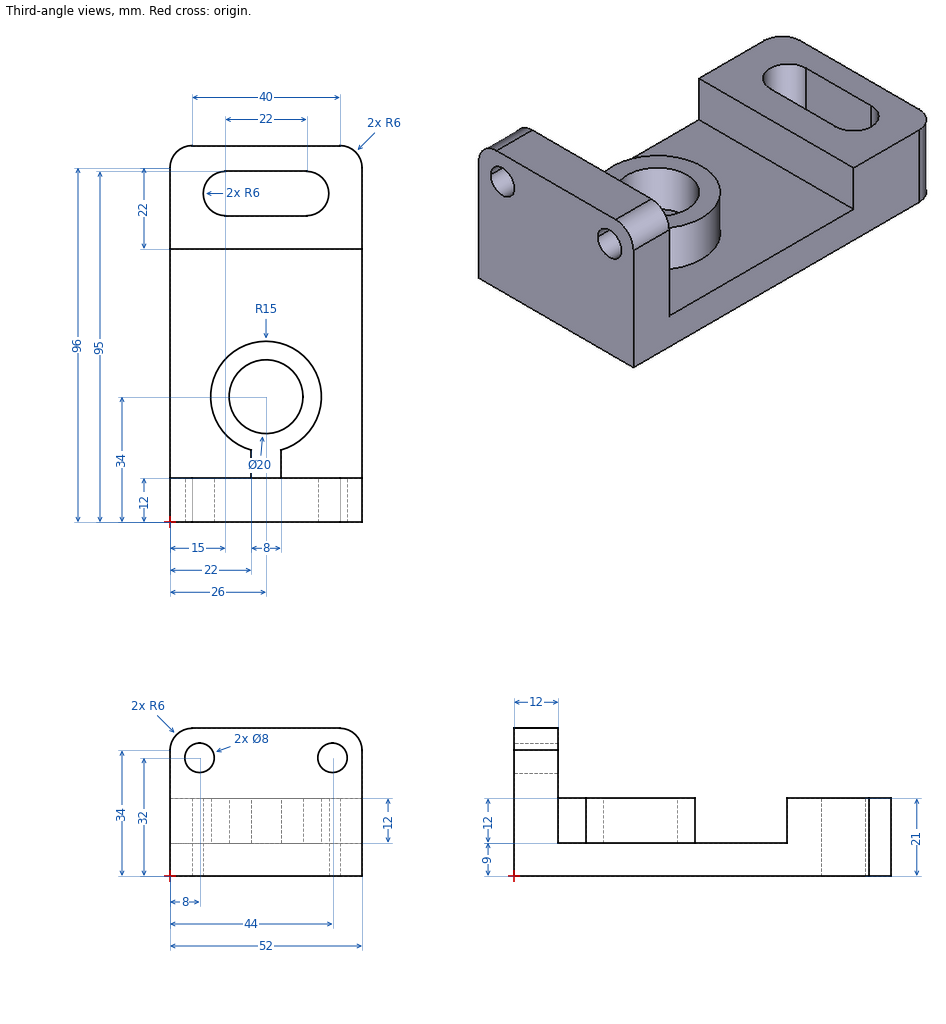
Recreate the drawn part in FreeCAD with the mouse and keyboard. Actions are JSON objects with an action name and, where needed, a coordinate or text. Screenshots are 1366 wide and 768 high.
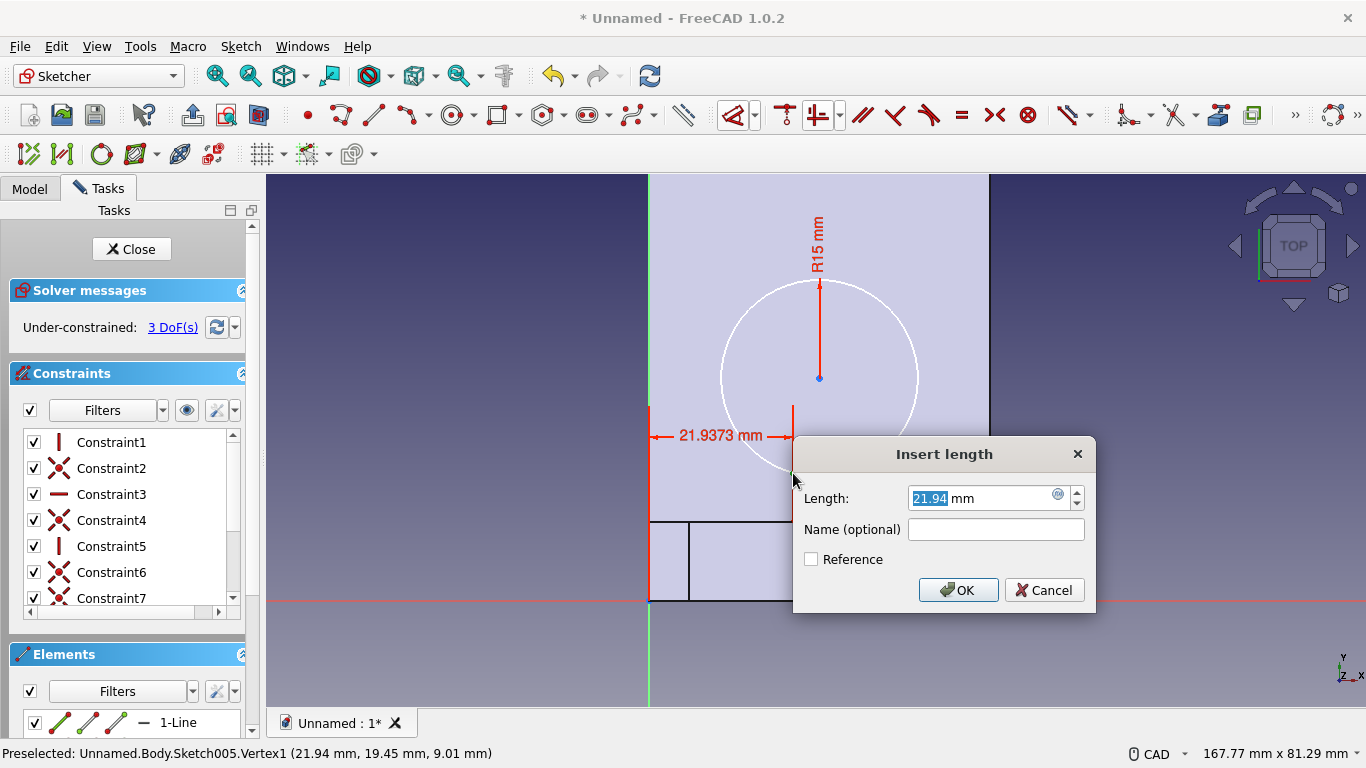
{"action": "type", "text": "22"}
{"action": "key", "text": "Return"}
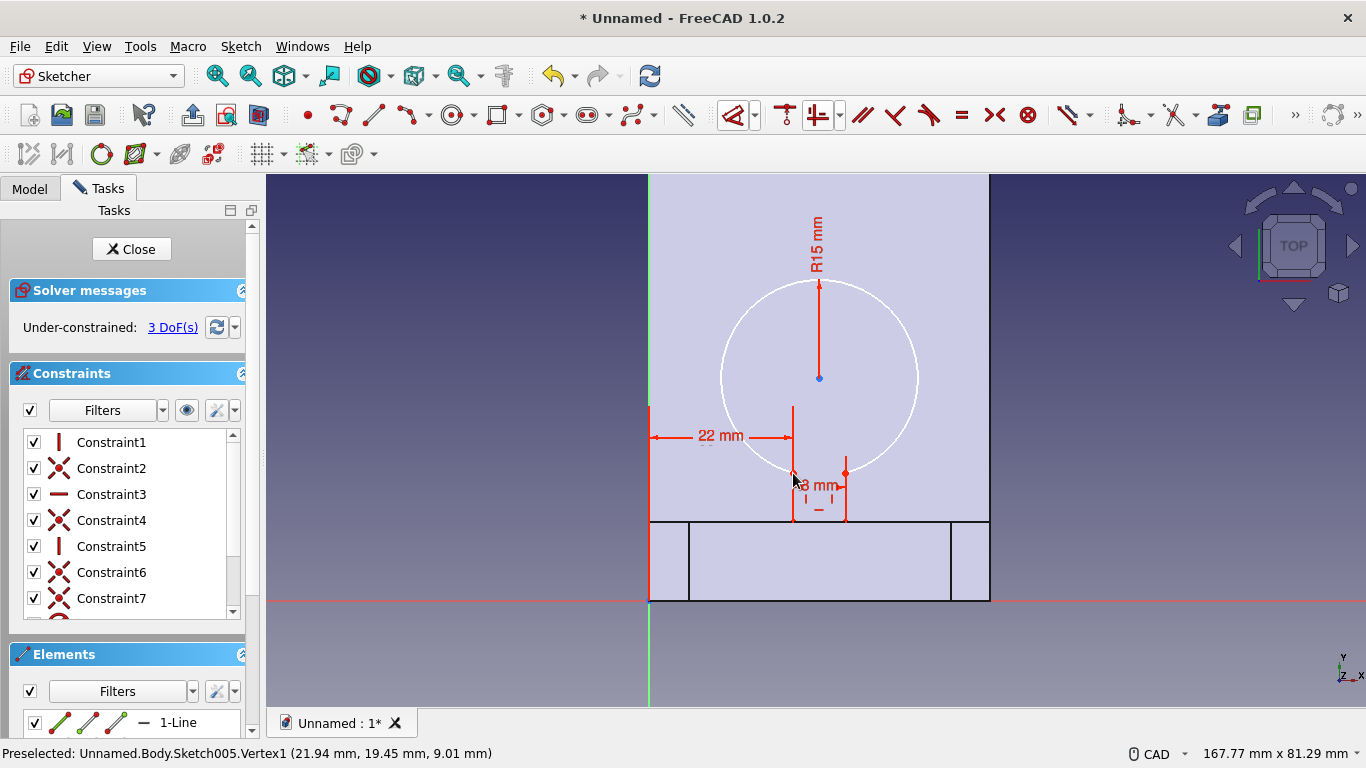
{"action": "left_click", "coordinate": [793, 523]}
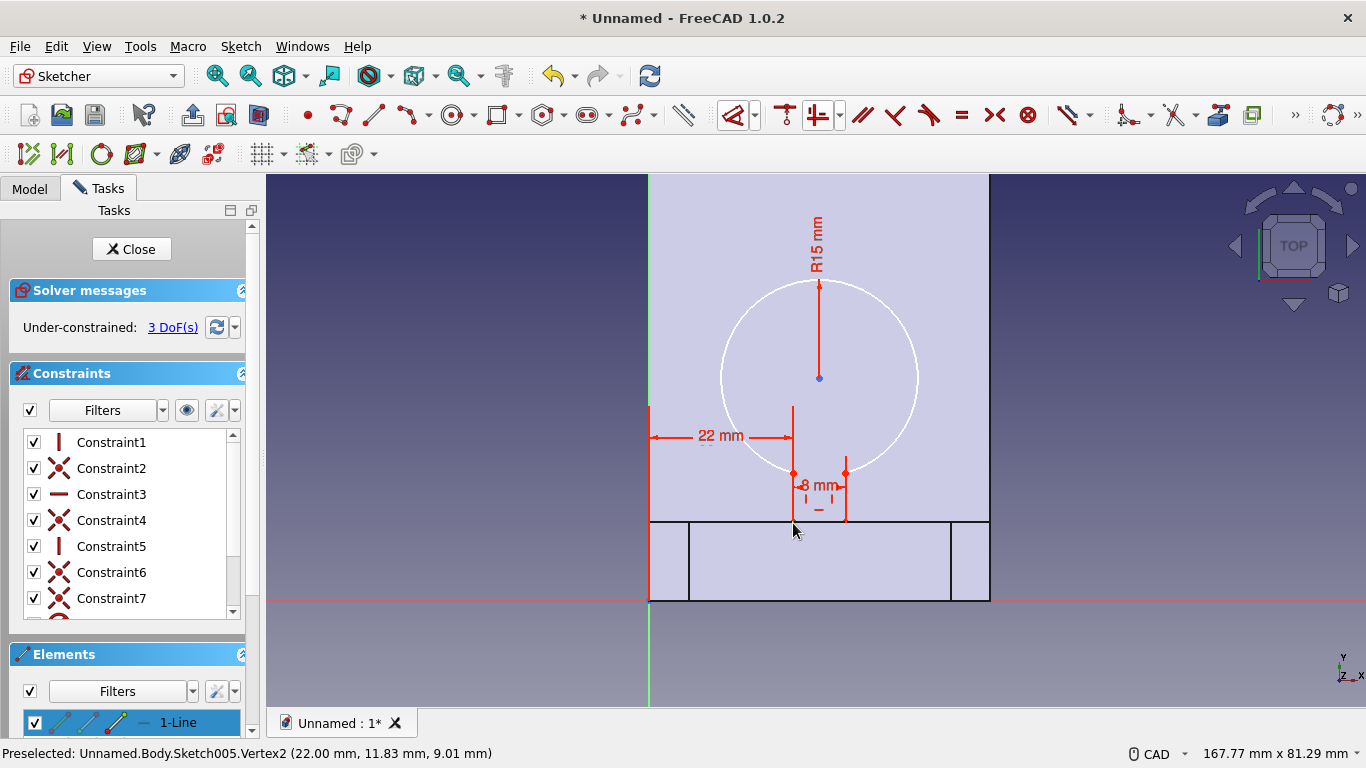
{"action": "left_click", "coordinate": [754, 116]}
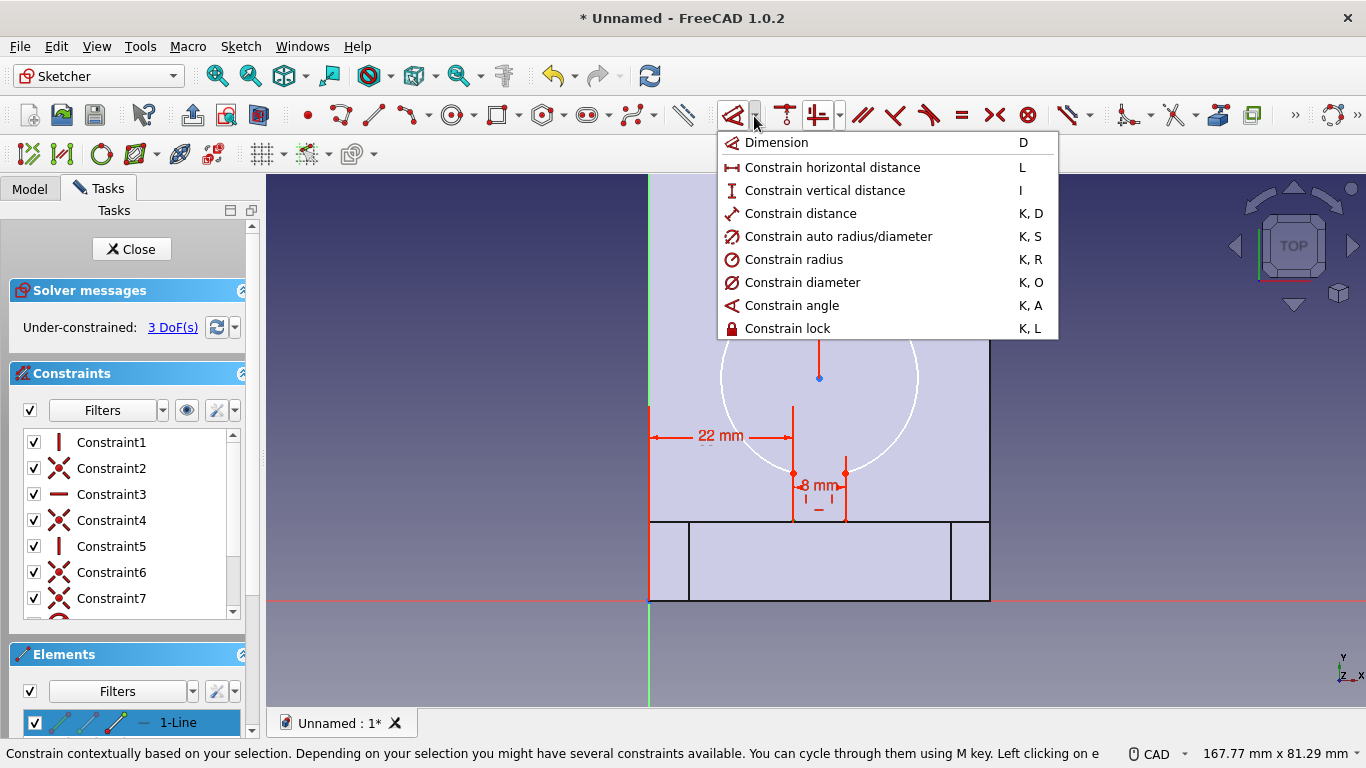
{"action": "left_click", "coordinate": [888, 190]}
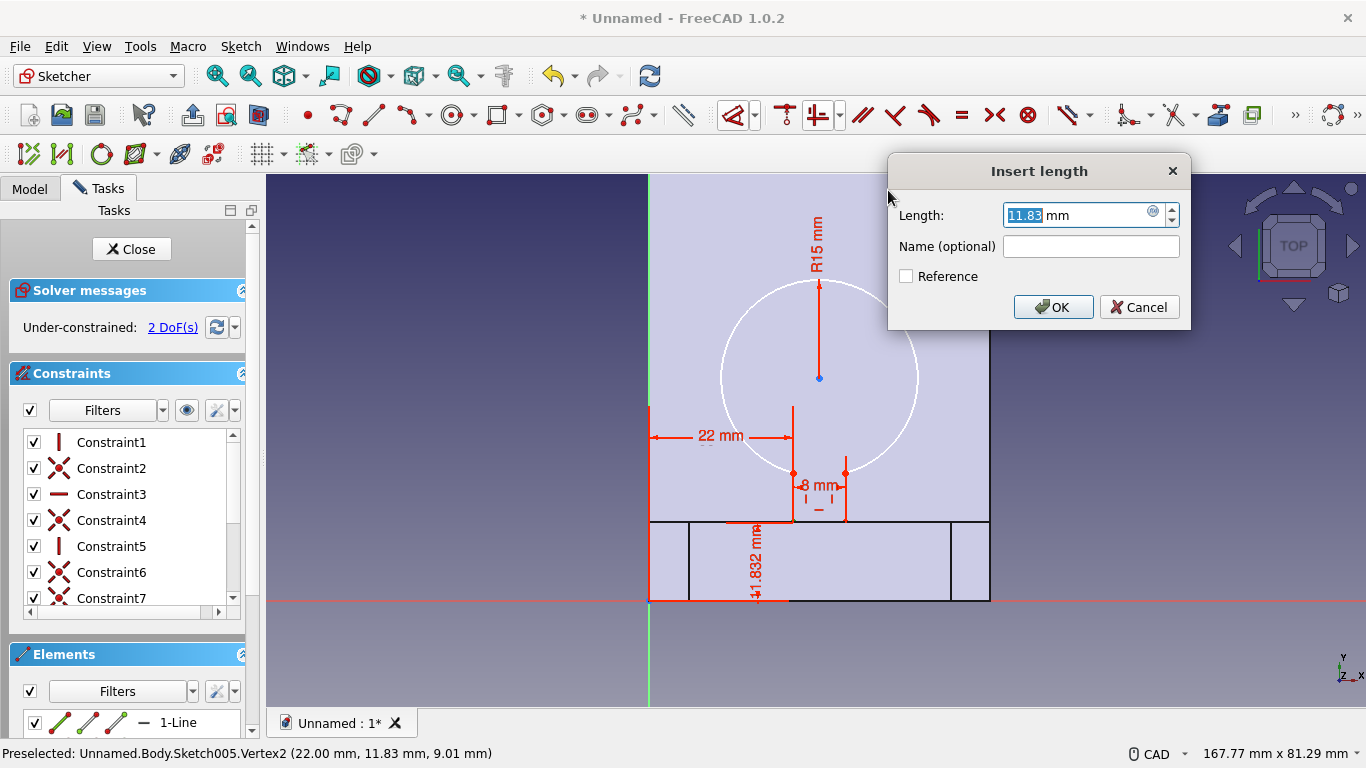
{"action": "type", "text": "12"}
{"action": "key", "text": "Return"}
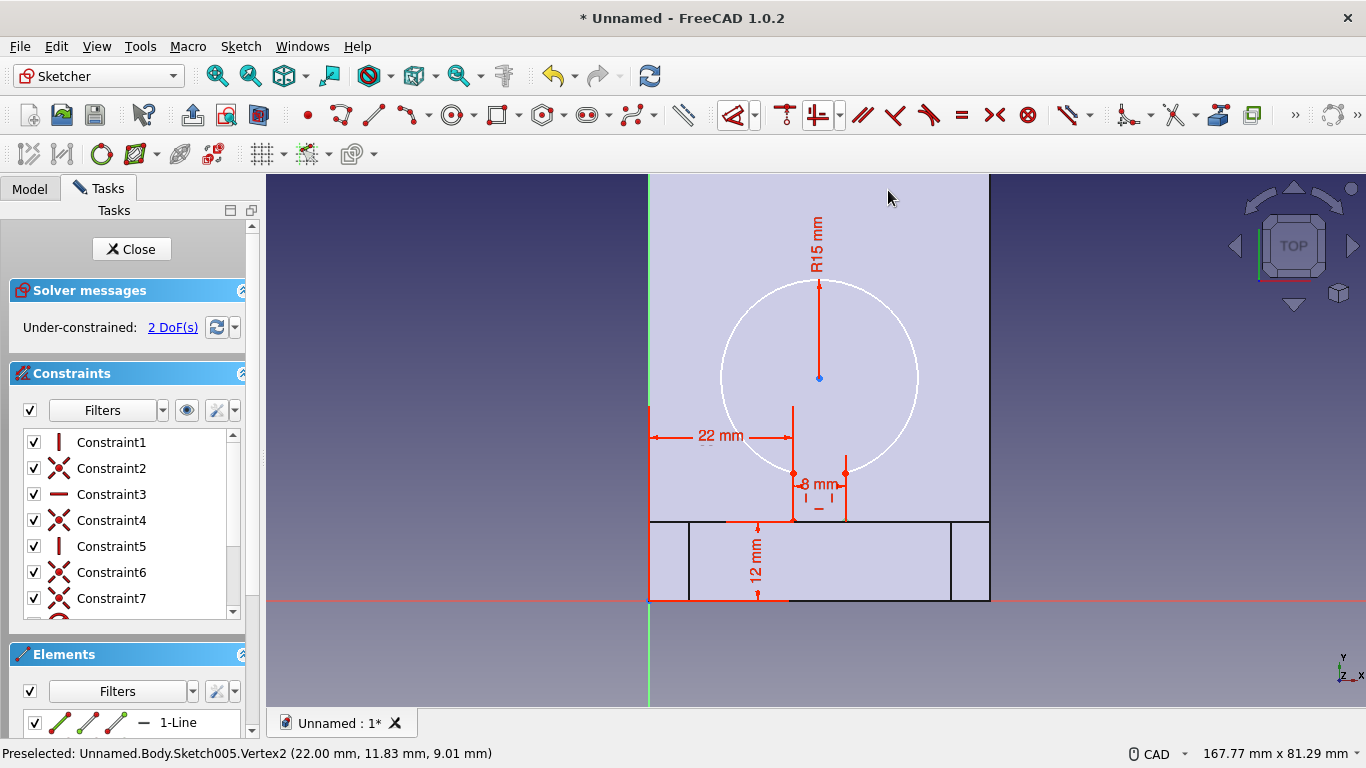
{"action": "left_click", "coordinate": [819, 378]}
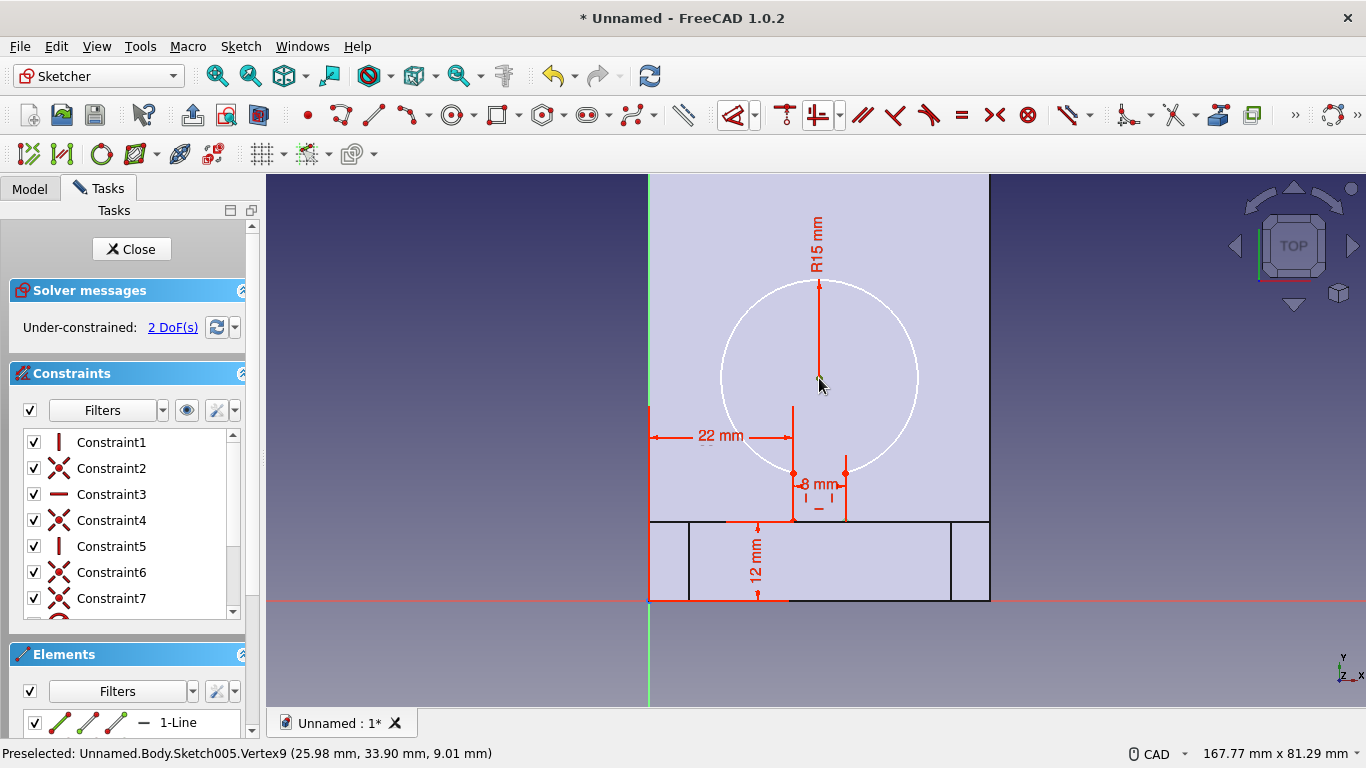
{"action": "key", "text": "l"}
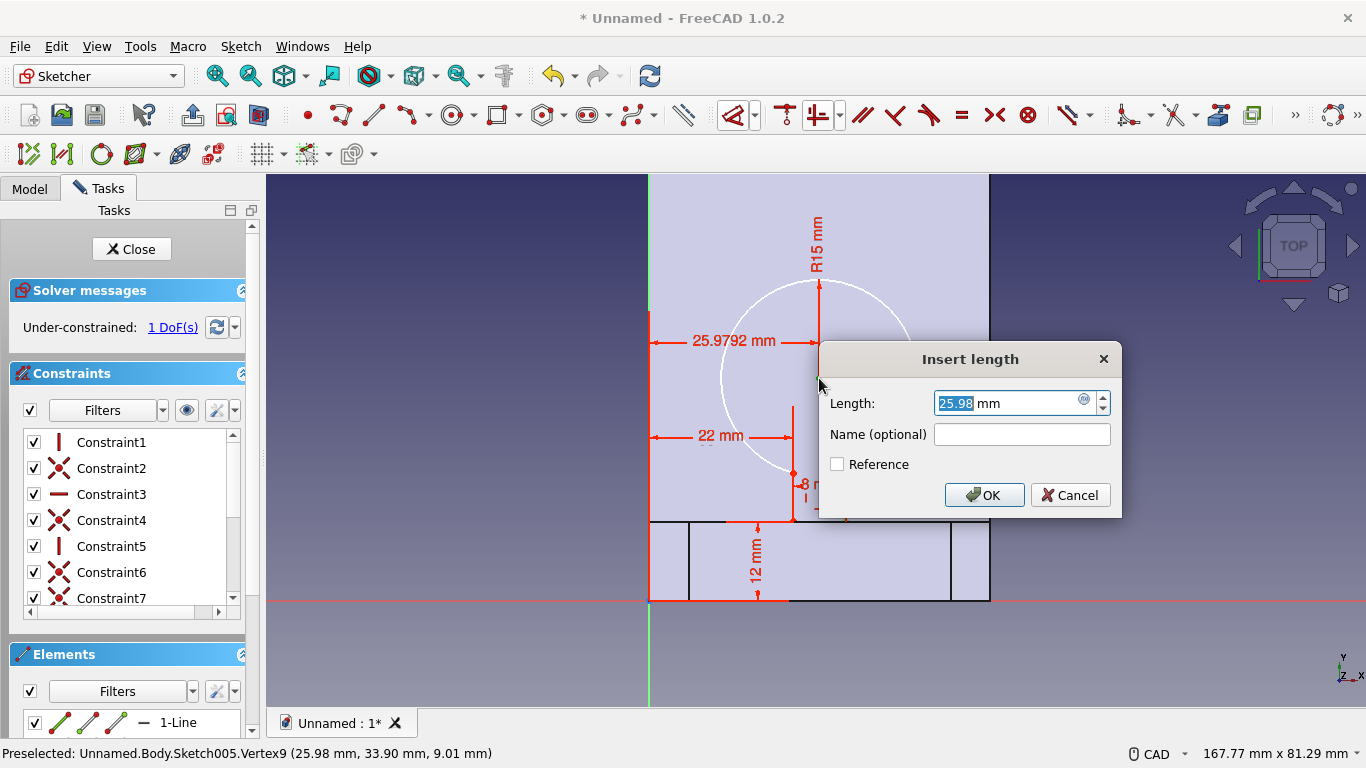
{"action": "type", "text": "26"}
{"action": "key", "text": "Return"}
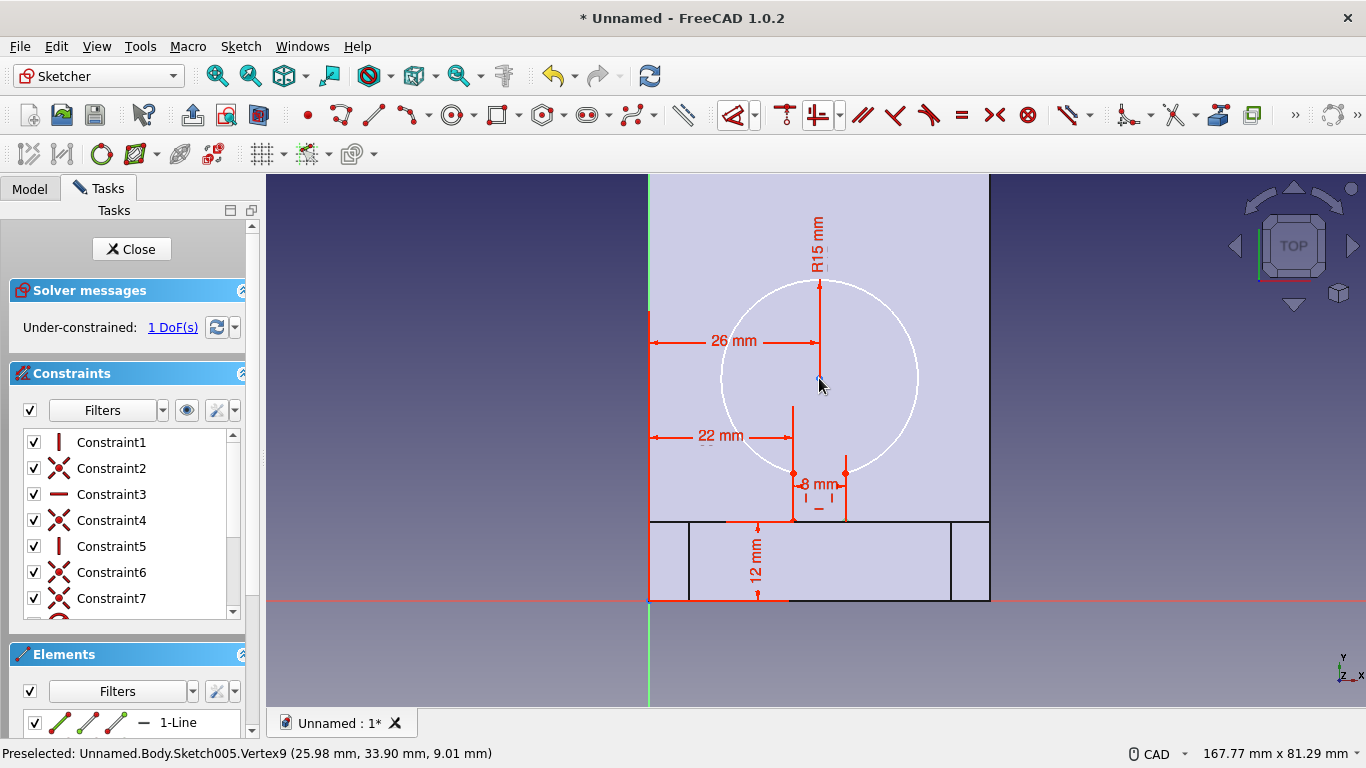
{"action": "left_click", "coordinate": [820, 378]}